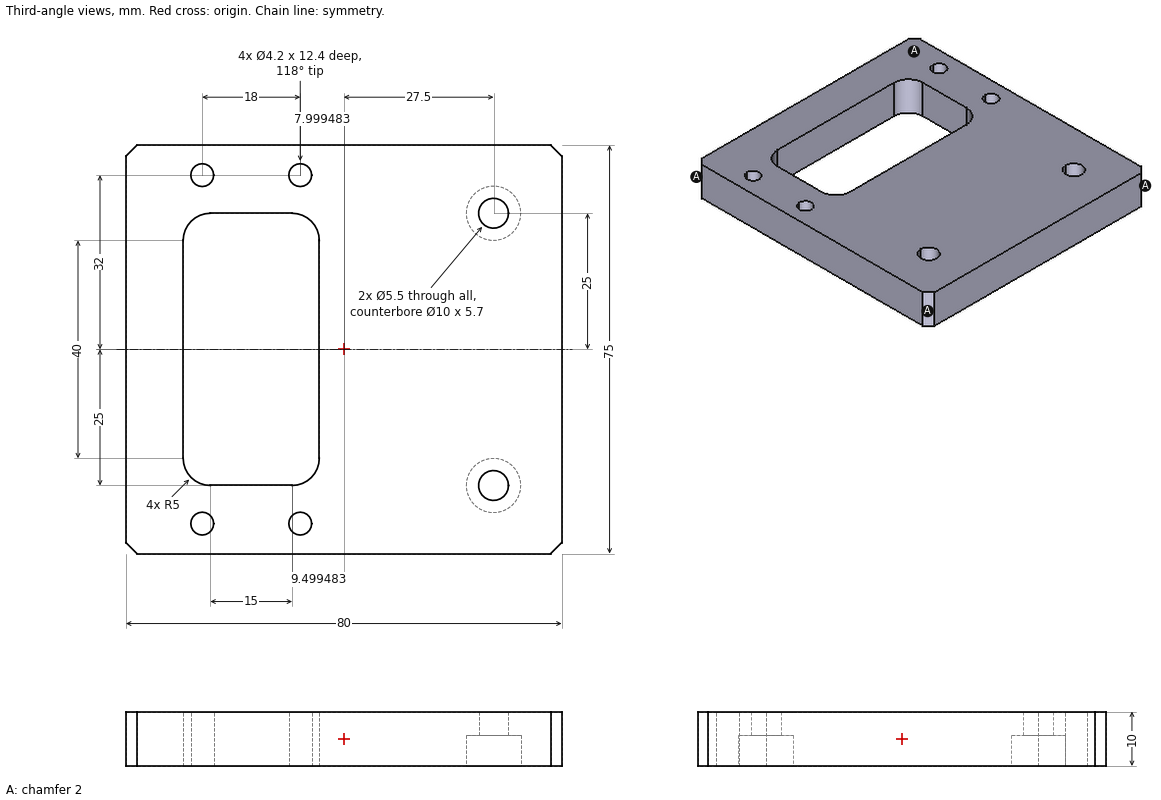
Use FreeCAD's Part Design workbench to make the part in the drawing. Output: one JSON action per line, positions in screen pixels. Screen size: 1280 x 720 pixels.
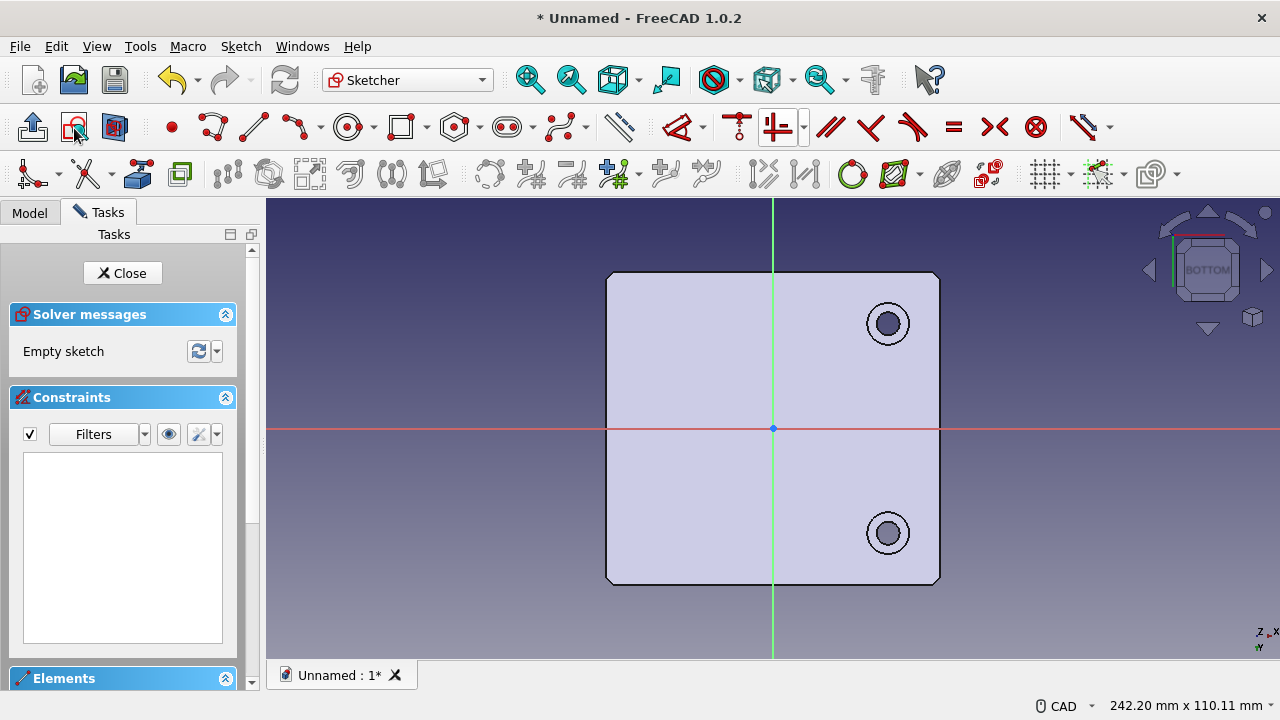
{"action": "key", "text": "g c"}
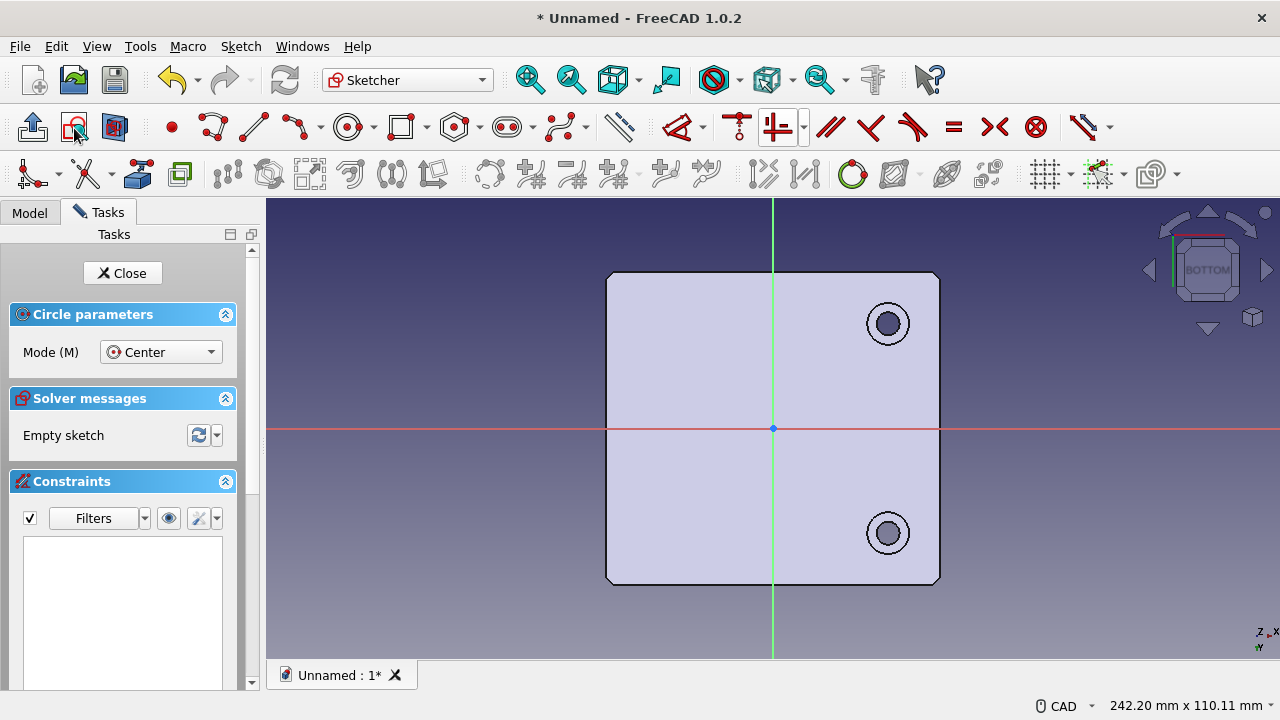
{"action": "scroll", "coordinate": [740, 562], "scroll_direction": "up", "scroll_amount": 5}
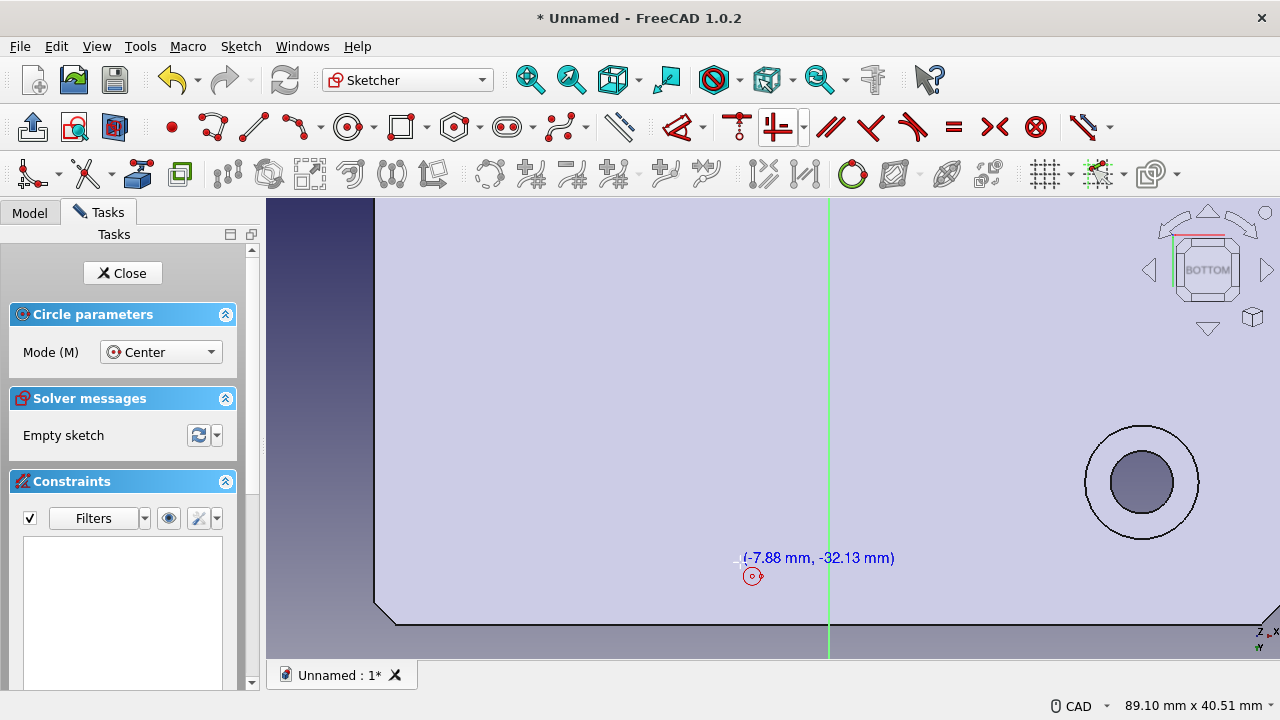
{"action": "left_click", "coordinate": [738, 562]}
{"action": "mouse_move", "coordinate": [755, 545]}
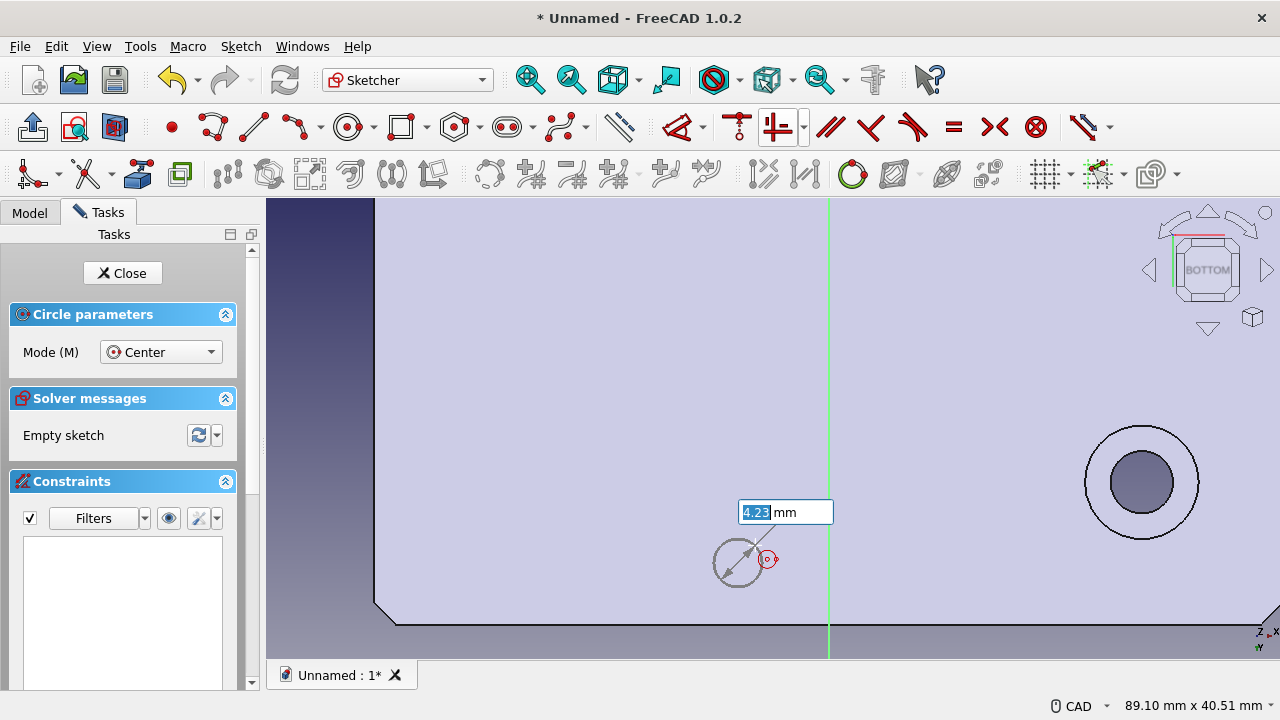
{"action": "type", "text": "4.2"}
{"action": "key", "text": "Return"}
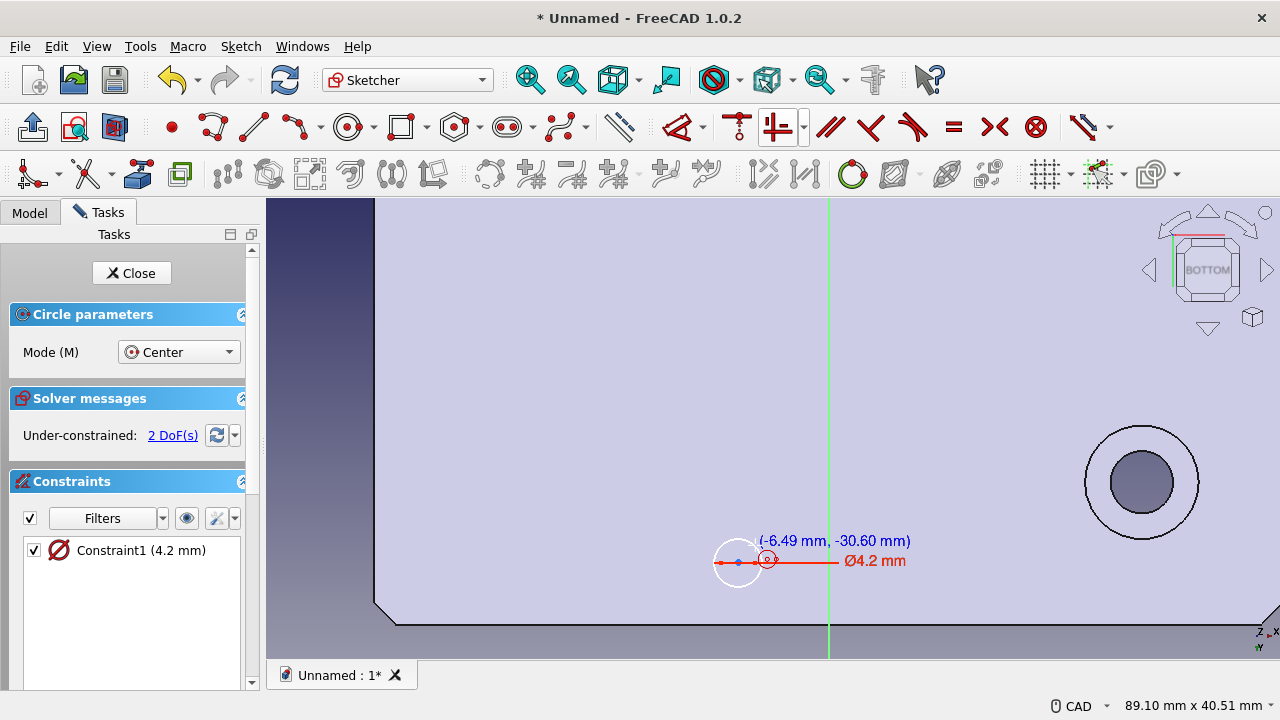
{"action": "left_click", "coordinate": [533, 562]}
{"action": "mouse_move", "coordinate": [550, 545]}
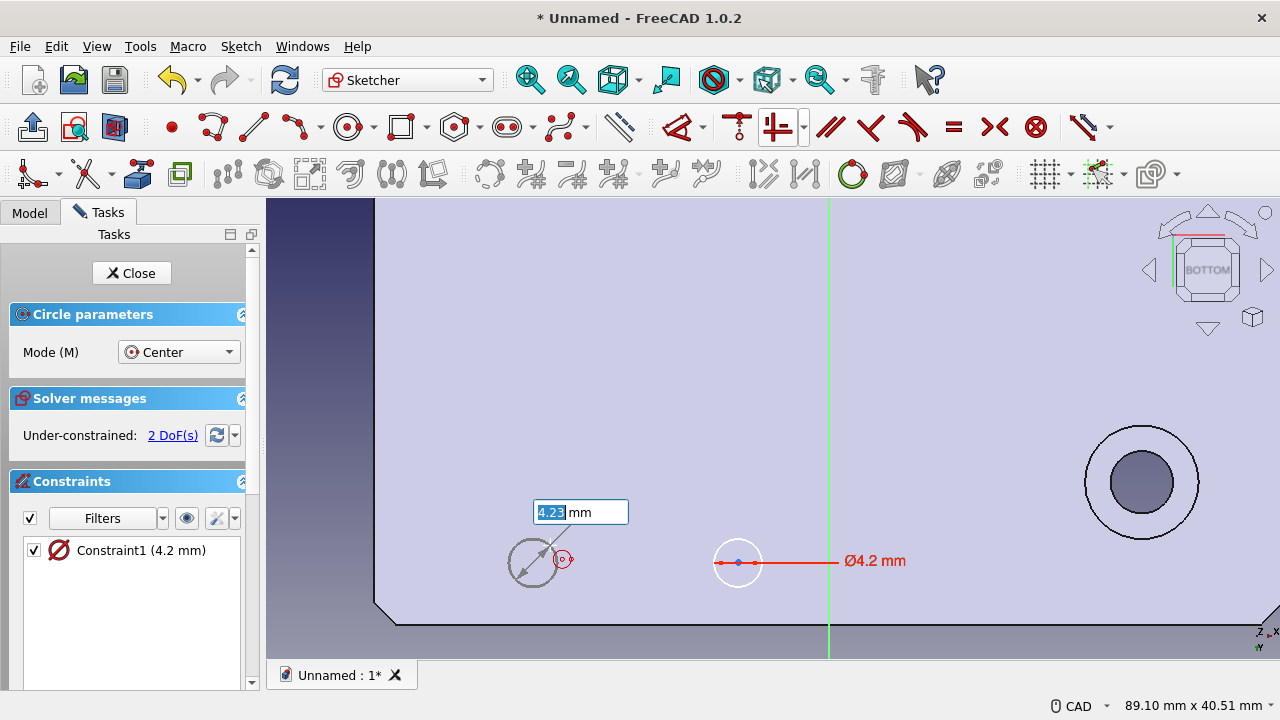
{"action": "type", "text": "4.2"}
{"action": "key", "text": "Return"}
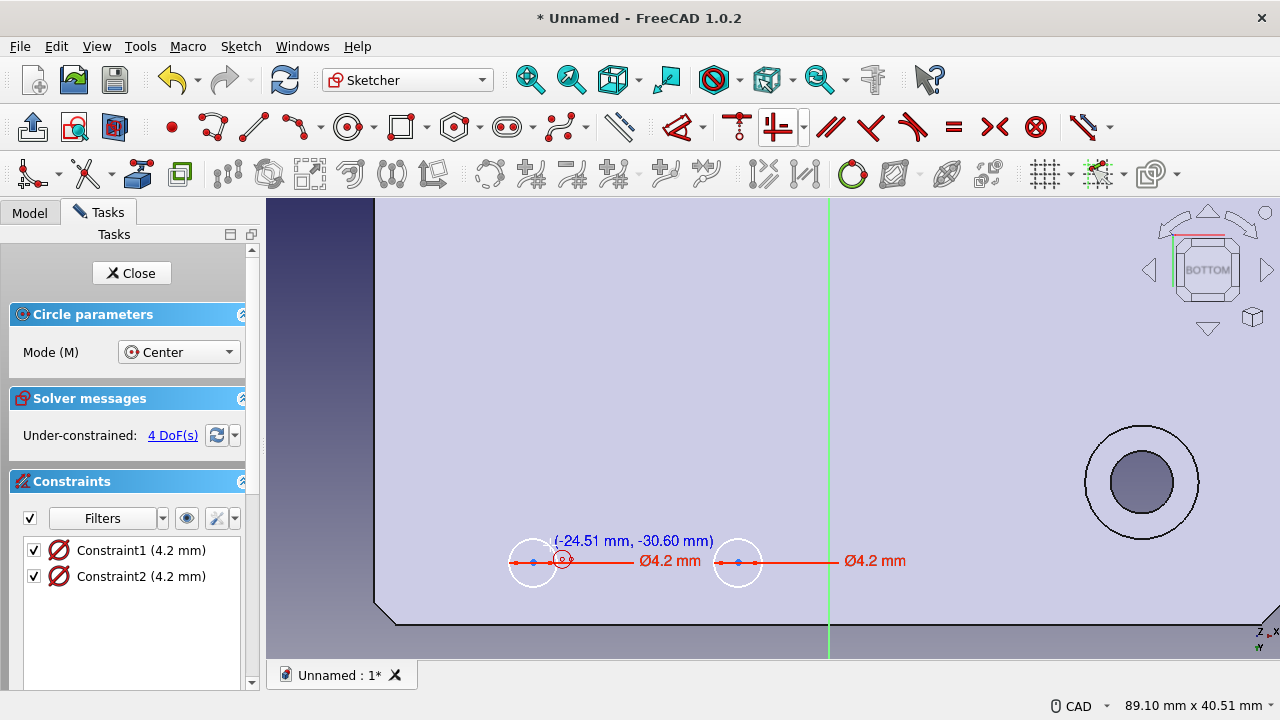
{"action": "scroll", "coordinate": [725, 563], "scroll_direction": "down", "scroll_amount": 5}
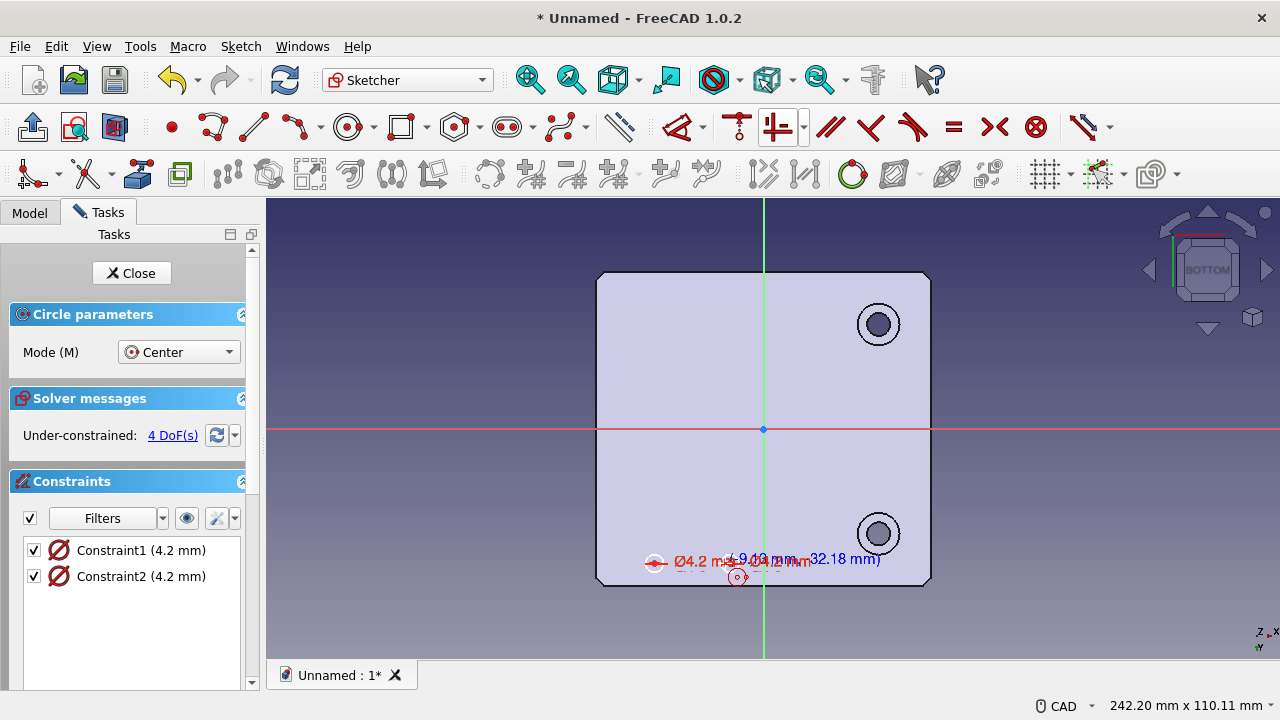
{"action": "scroll", "coordinate": [730, 295], "scroll_direction": "up", "scroll_amount": 5}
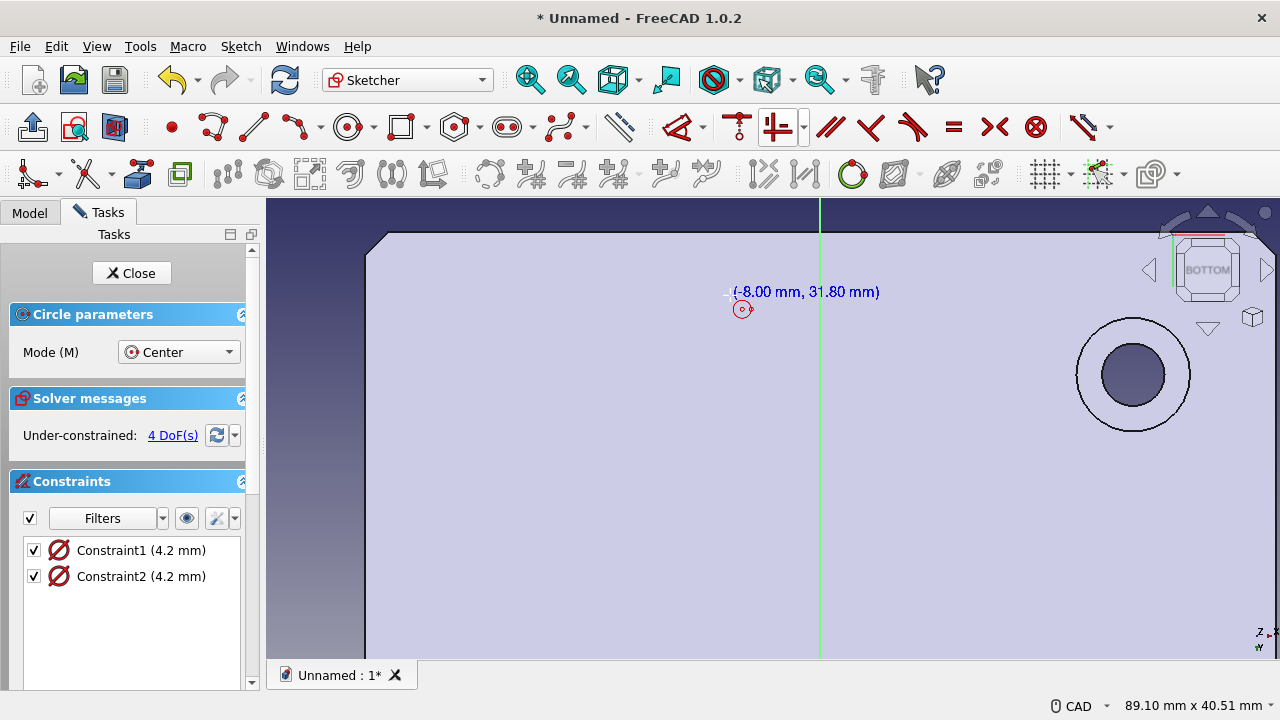
{"action": "left_click", "coordinate": [729, 295]}
{"action": "mouse_move", "coordinate": [746, 278]}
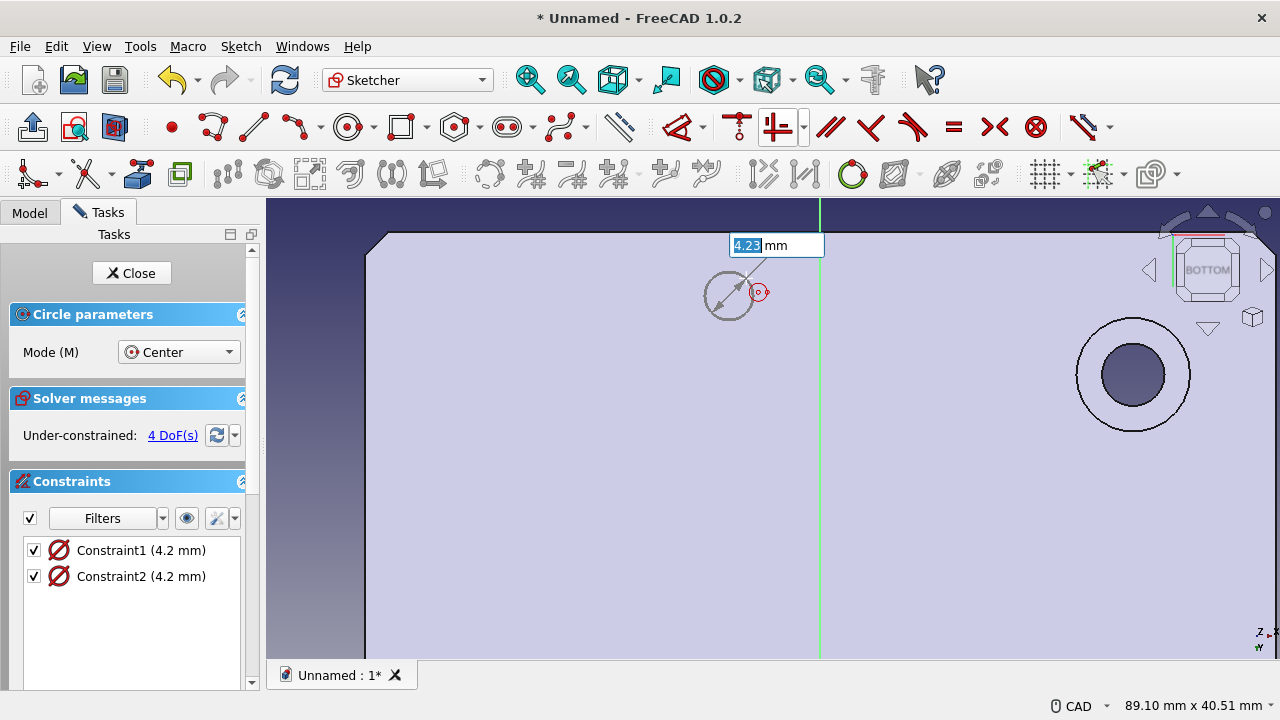
{"action": "type", "text": "4.2"}
{"action": "key", "text": "Return"}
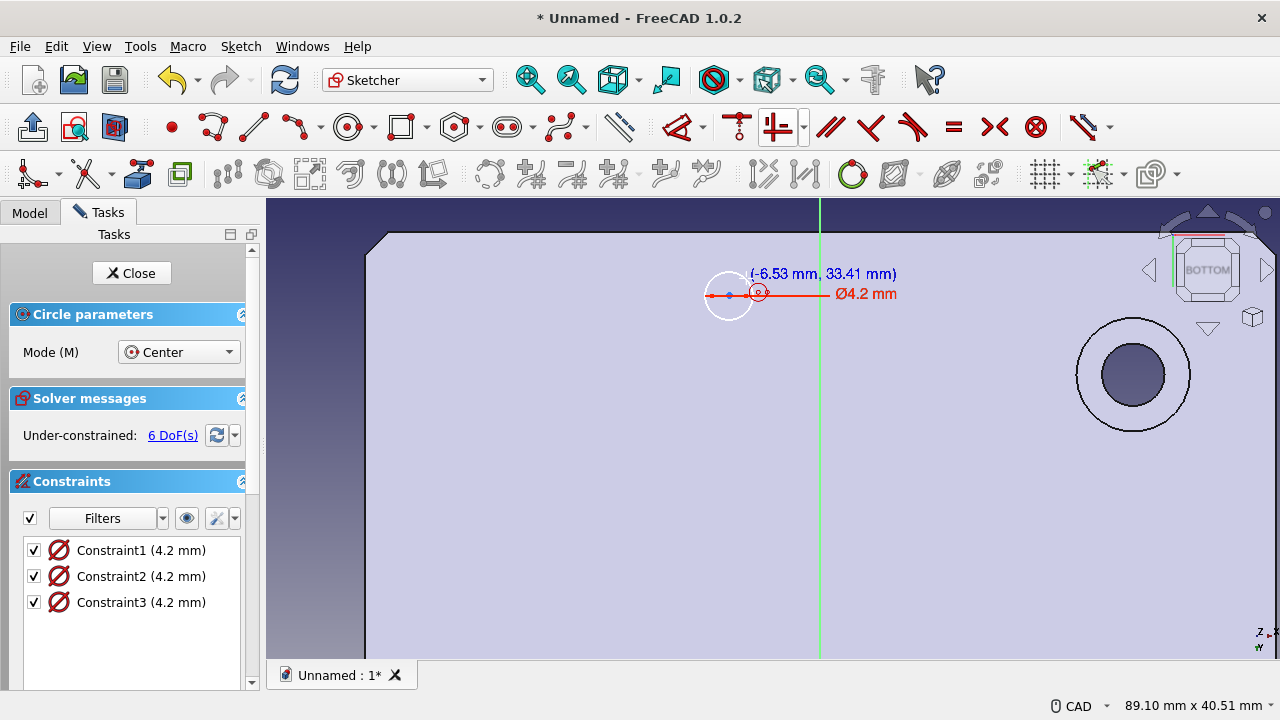
{"action": "left_click", "coordinate": [524, 295]}
{"action": "mouse_move", "coordinate": [541, 278]}